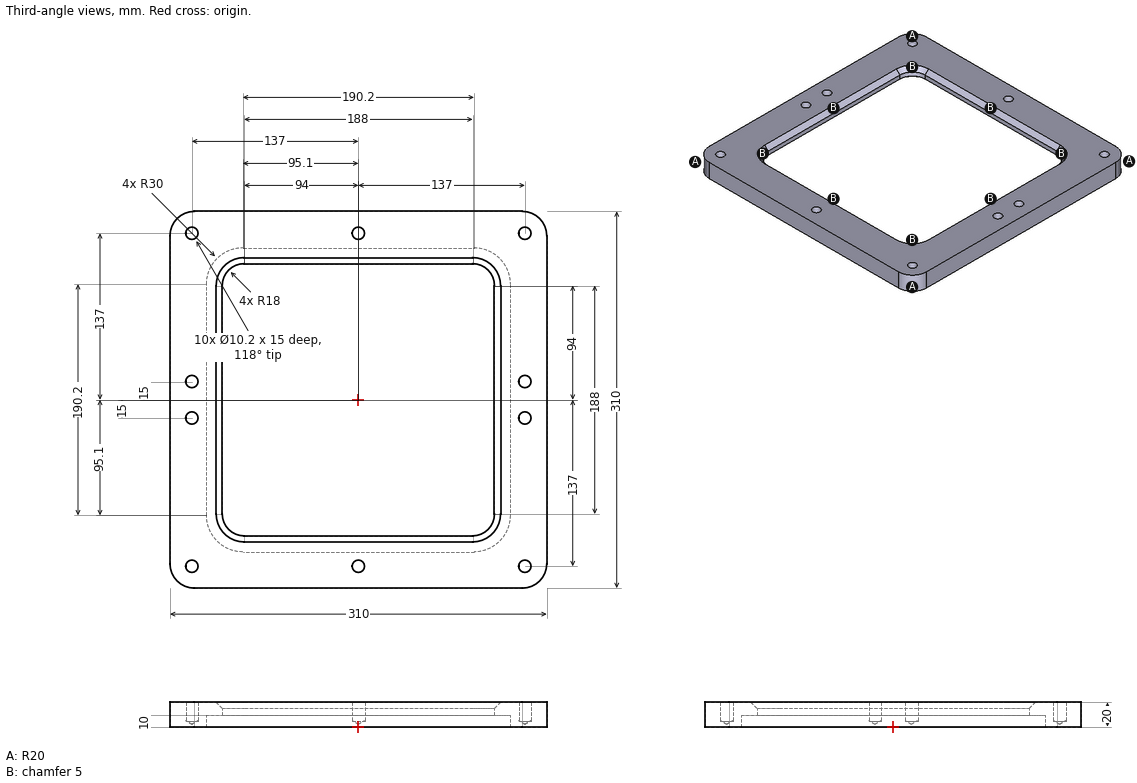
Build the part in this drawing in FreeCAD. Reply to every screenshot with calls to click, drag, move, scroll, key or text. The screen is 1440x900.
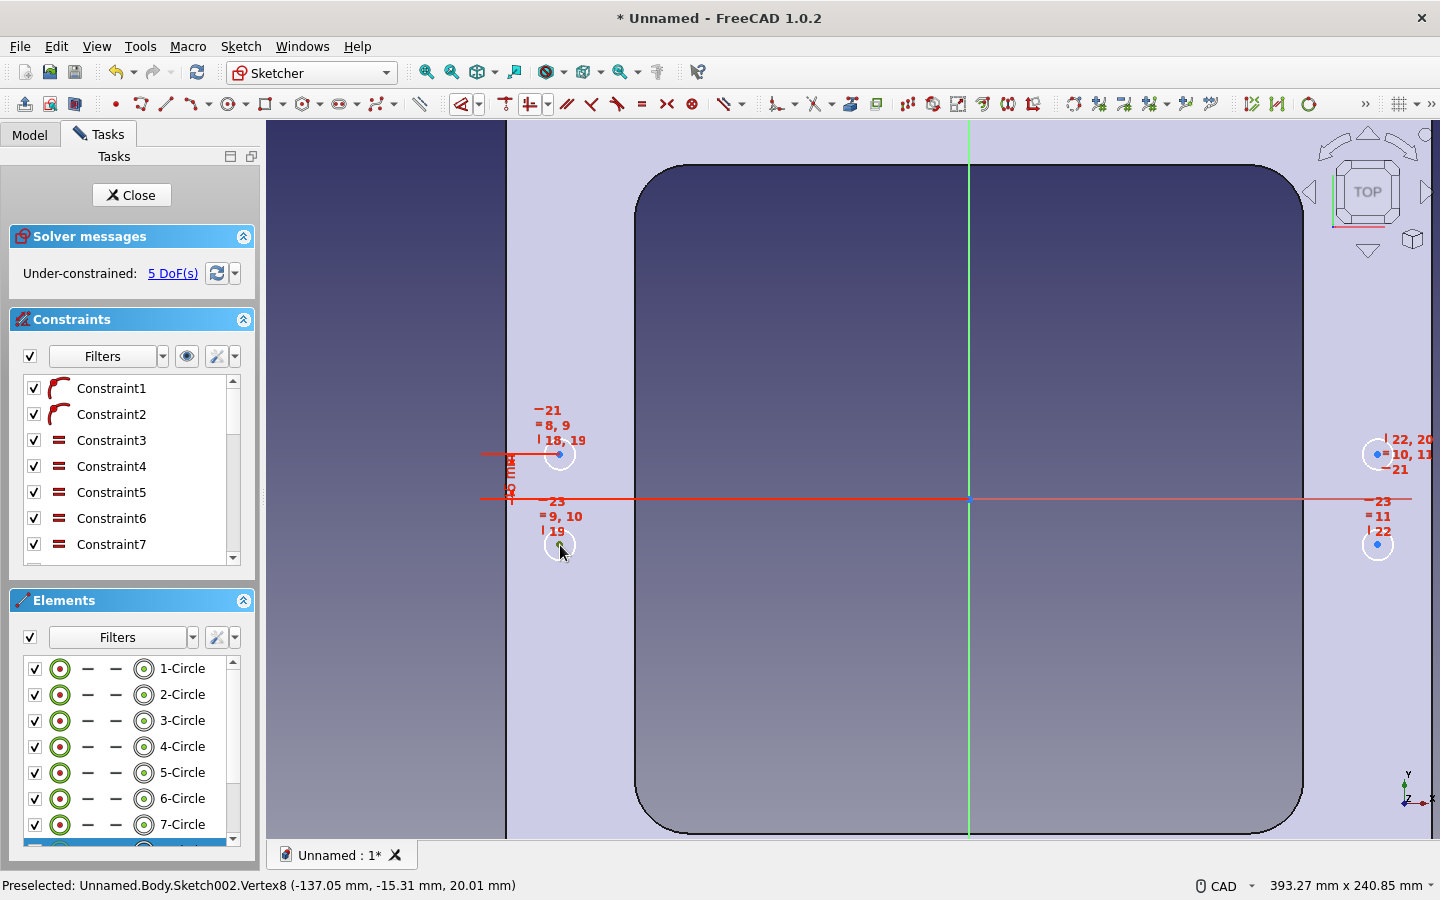
click(478, 104)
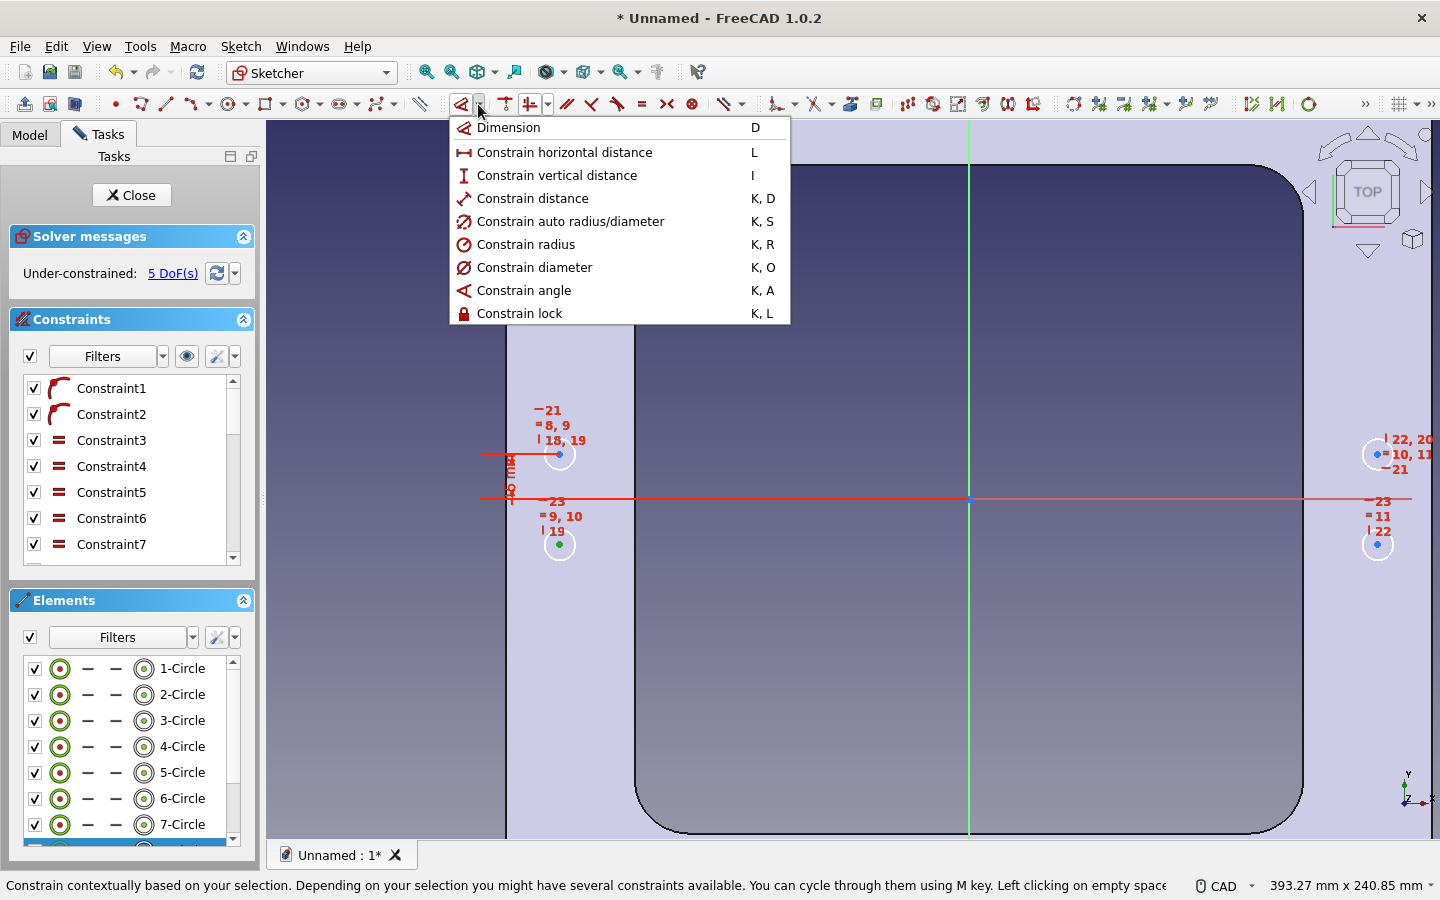
click(620, 176)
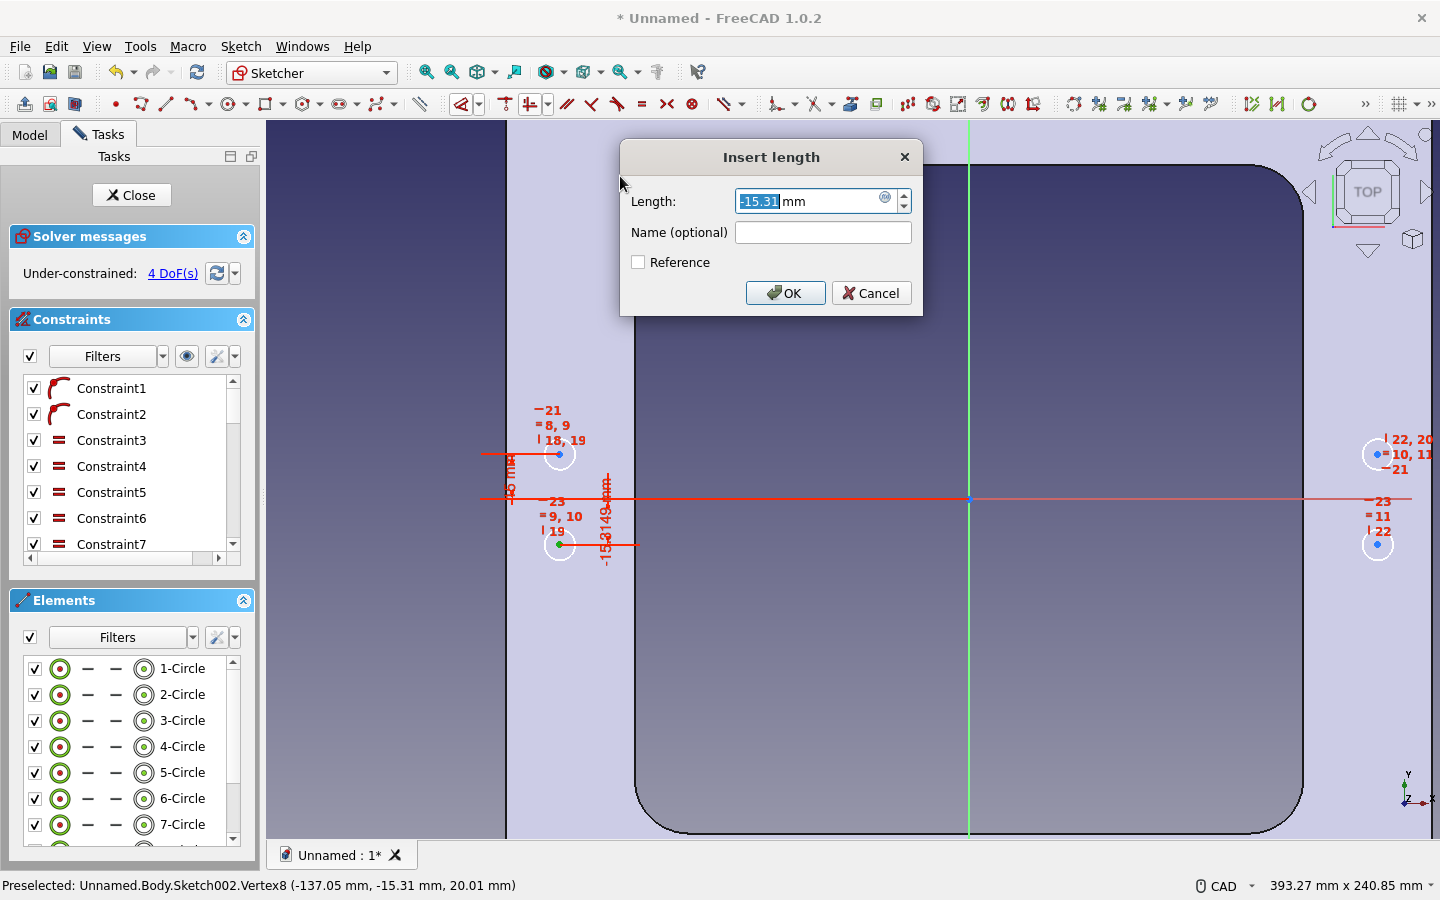
text(-15)
key(Return)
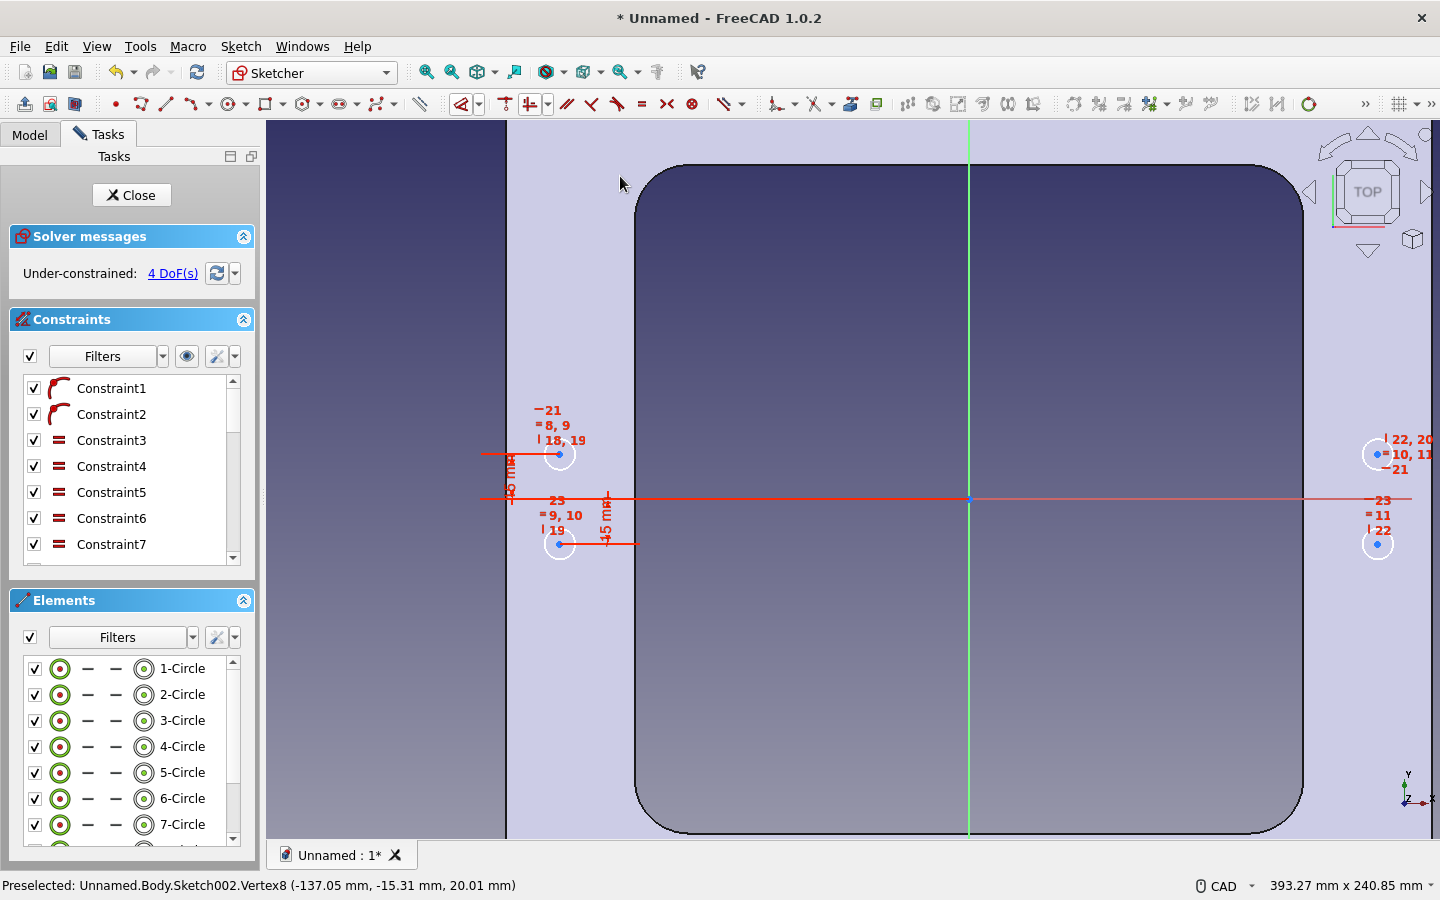
scroll(560, 455, down, 3)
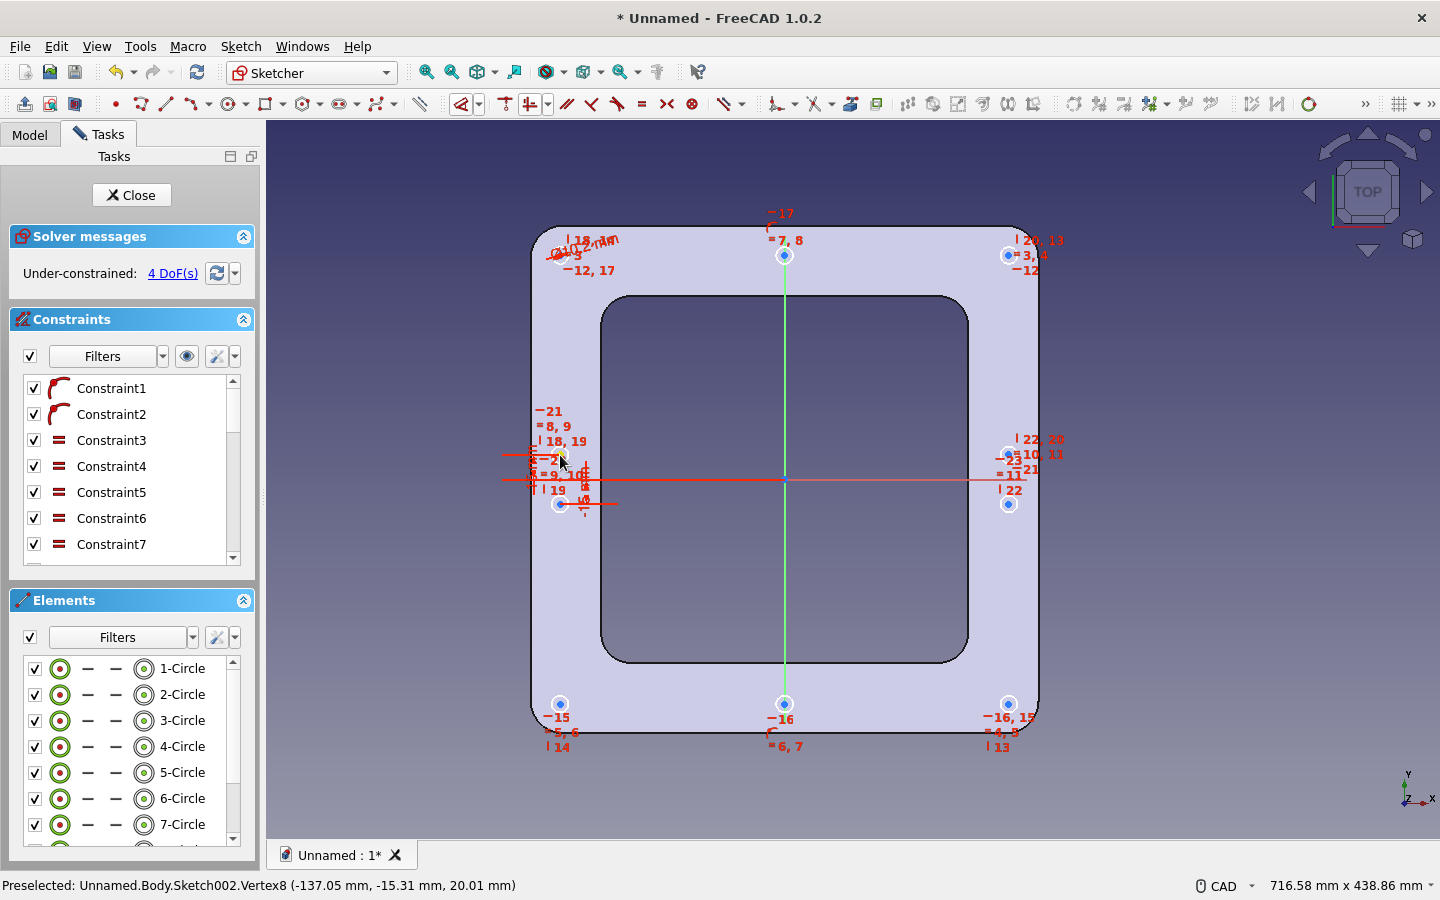
click(560, 255)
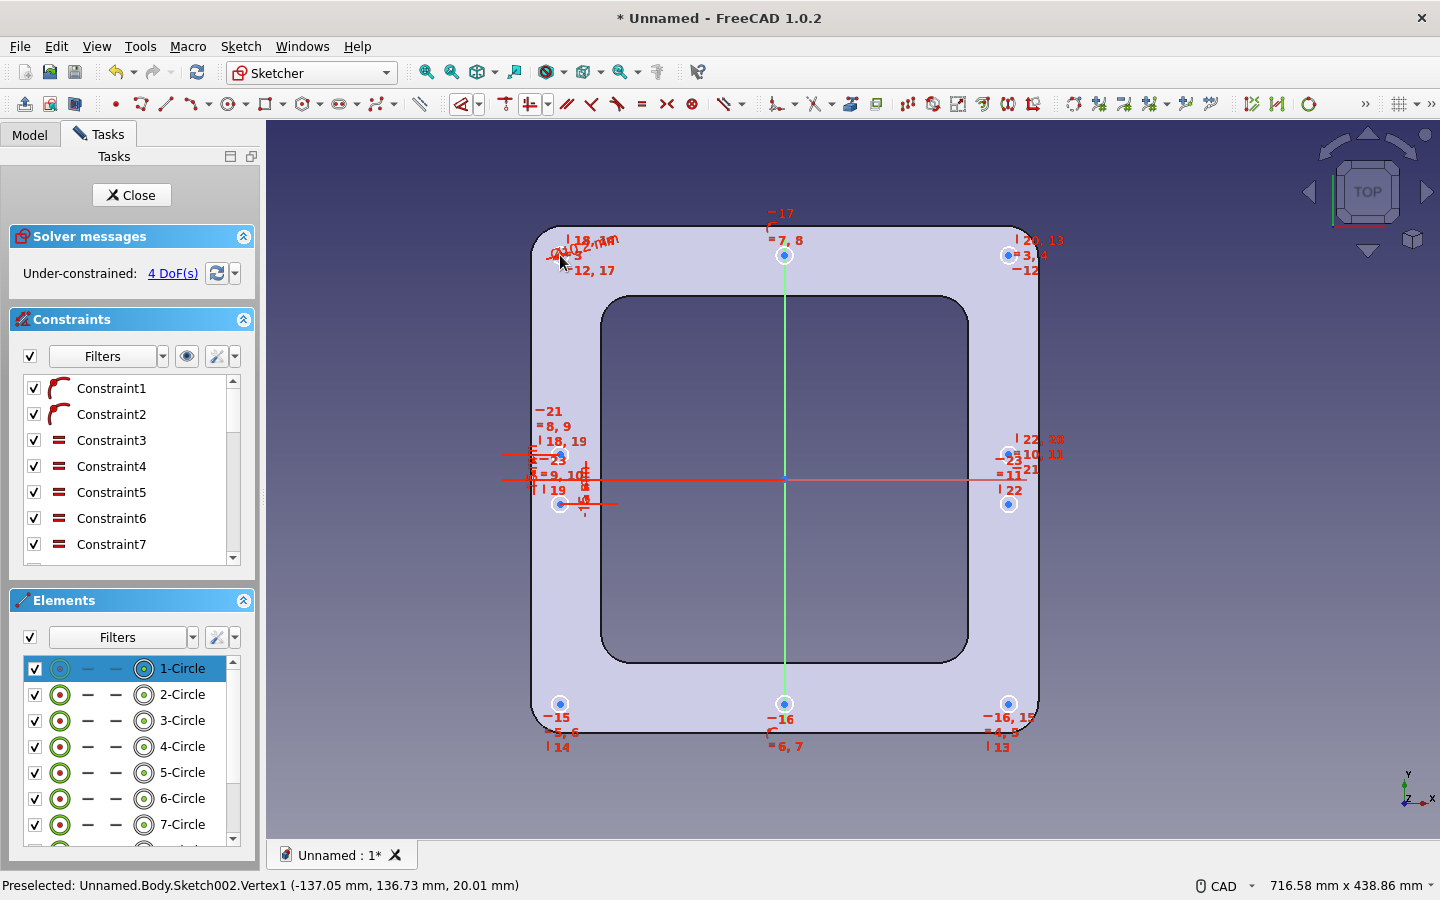
click(478, 104)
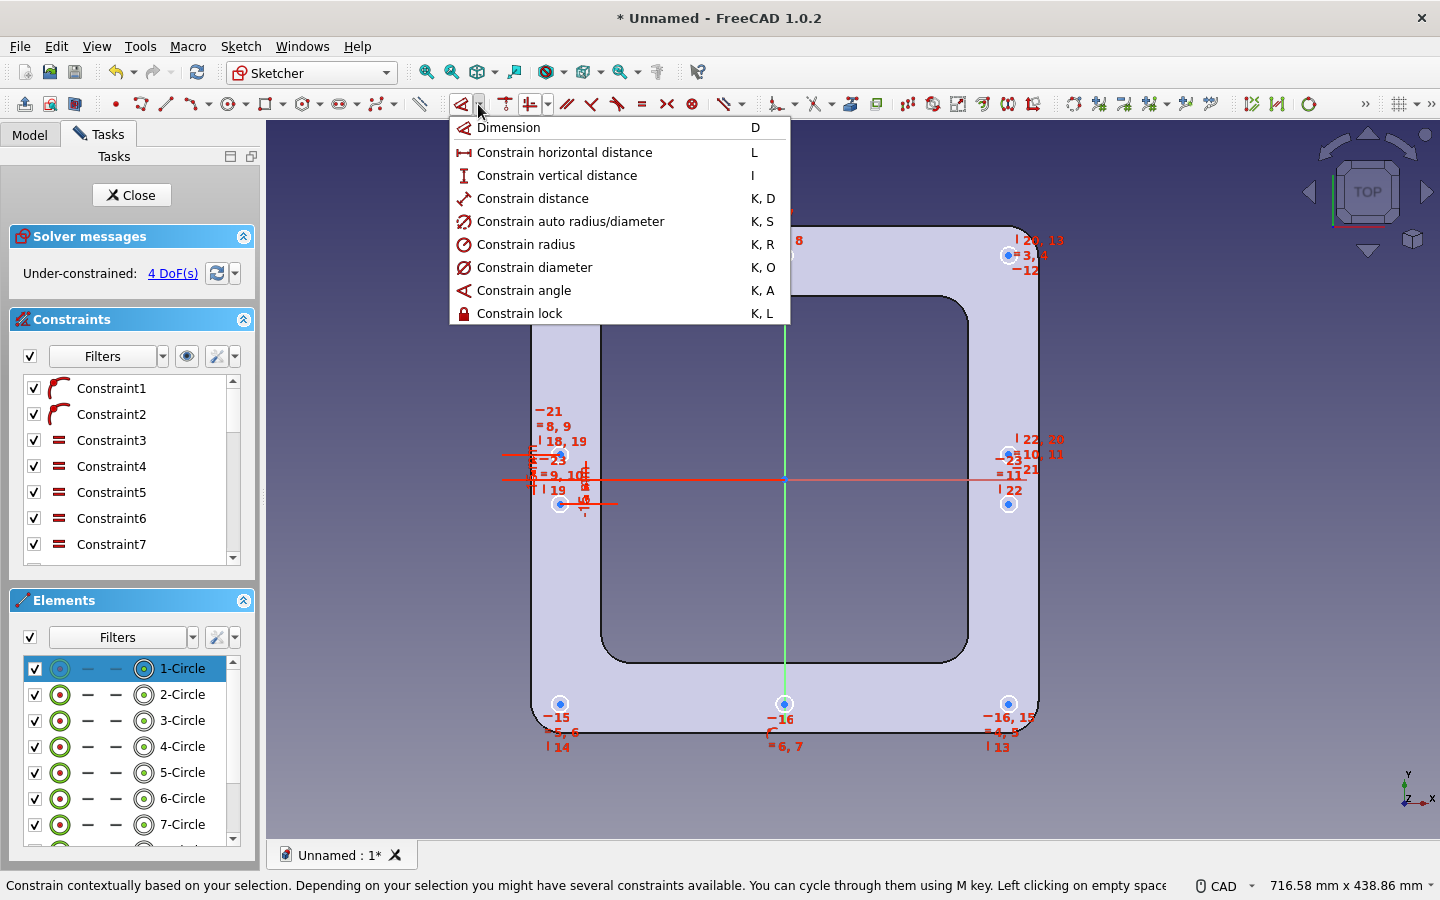
click(620, 152)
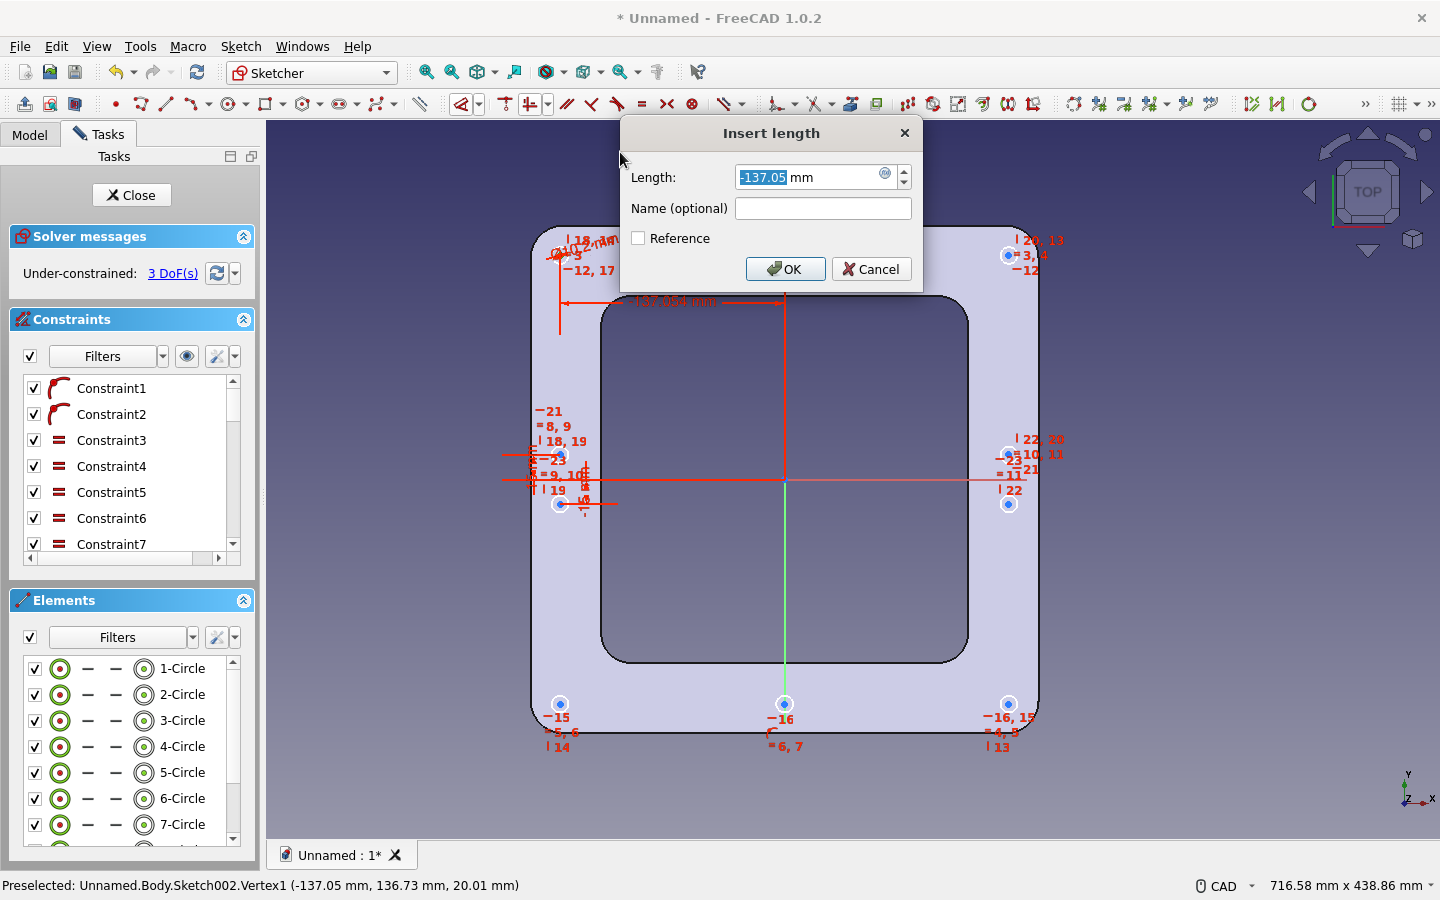
text(-137)
key(Return)